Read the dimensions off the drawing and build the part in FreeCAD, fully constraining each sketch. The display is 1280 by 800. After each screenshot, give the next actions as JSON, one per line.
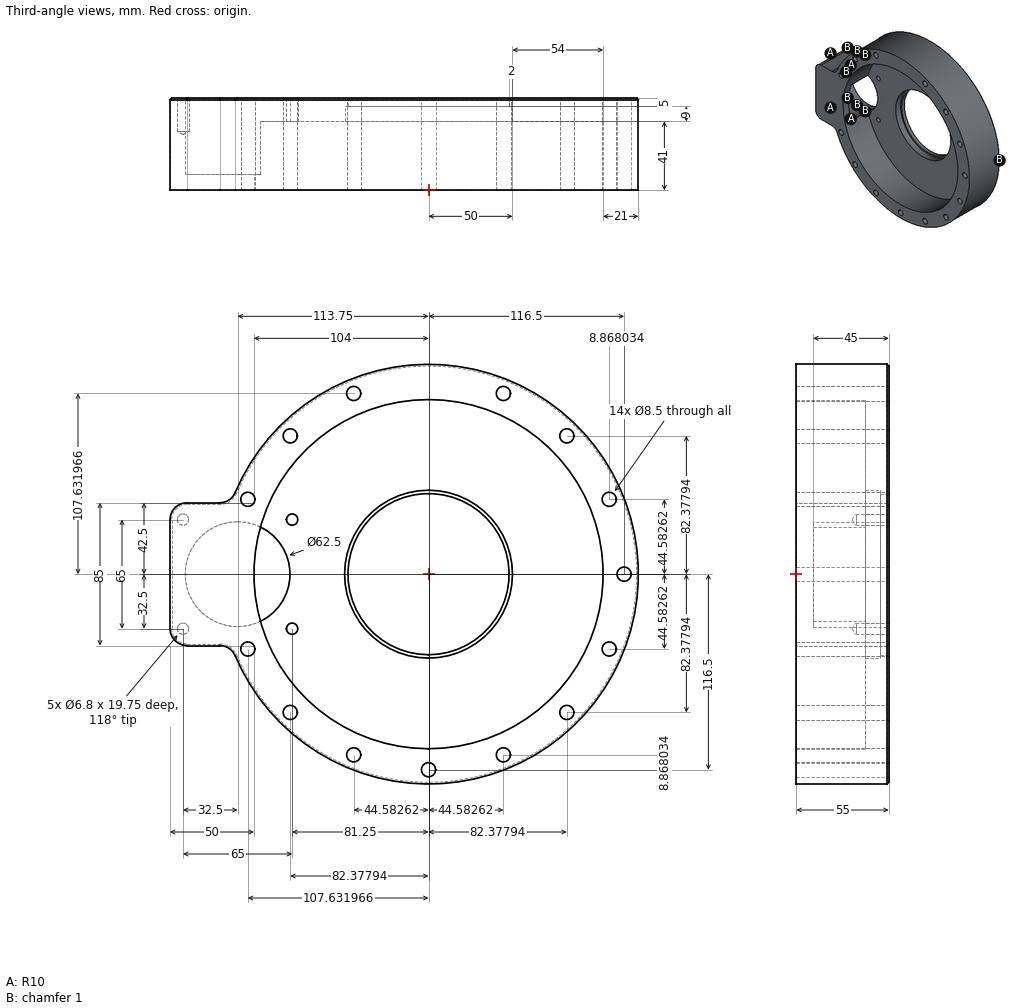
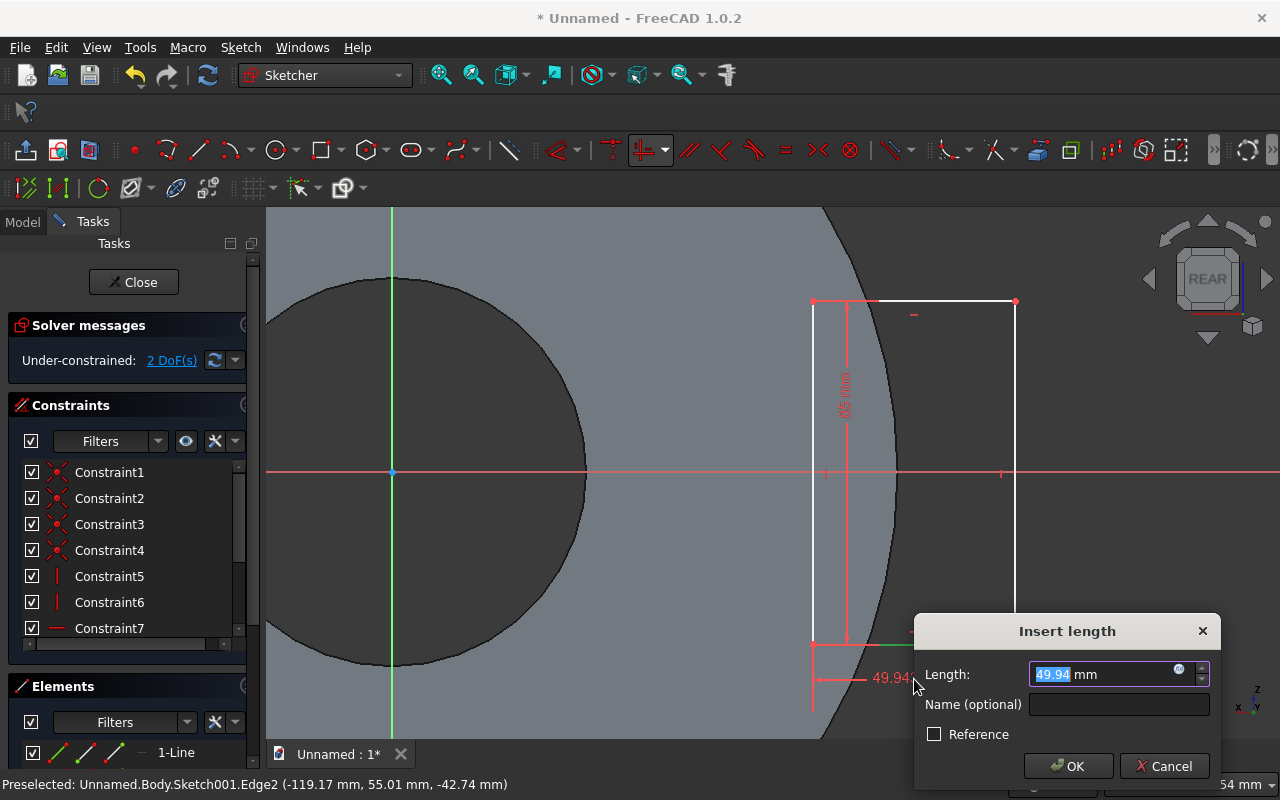
{"action": "type", "text": "50"}
{"action": "key", "text": "Return"}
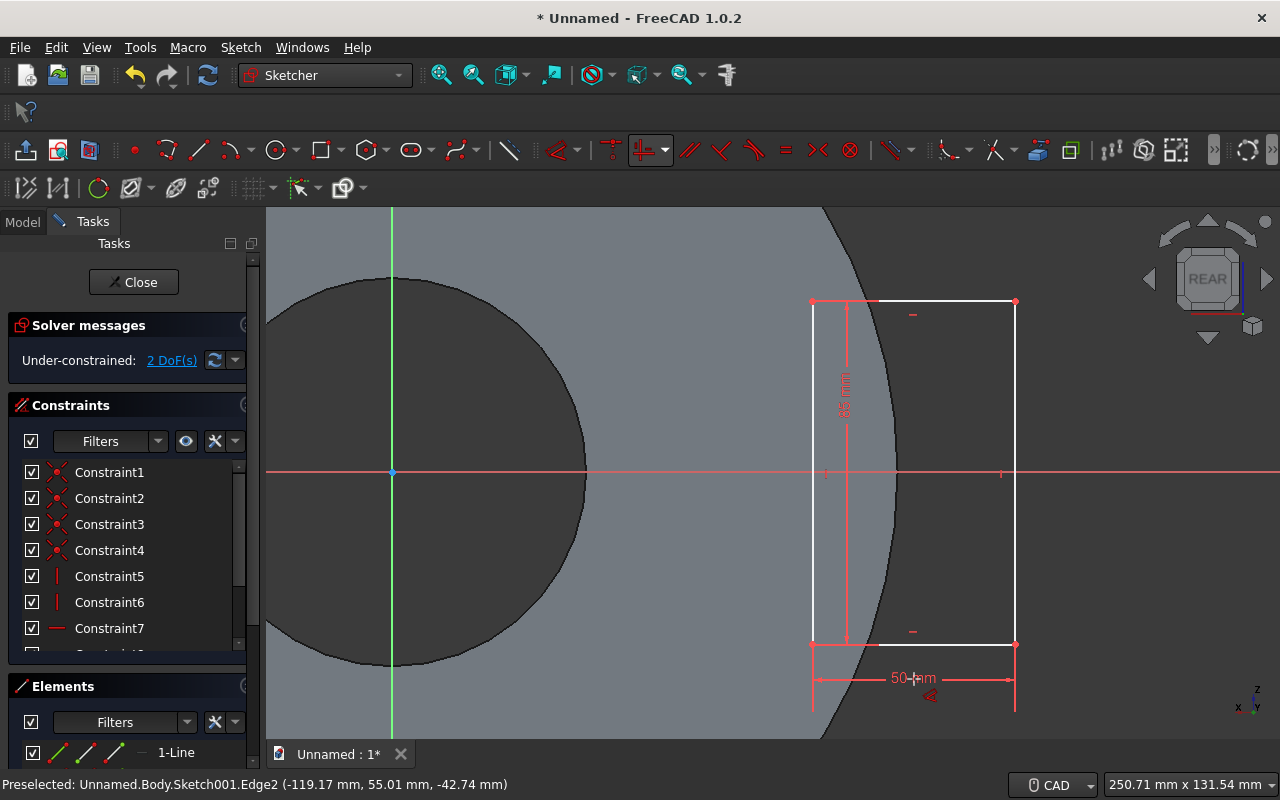
{"action": "left_click", "coordinate": [813, 301]}
{"action": "left_click", "coordinate": [602, 267]}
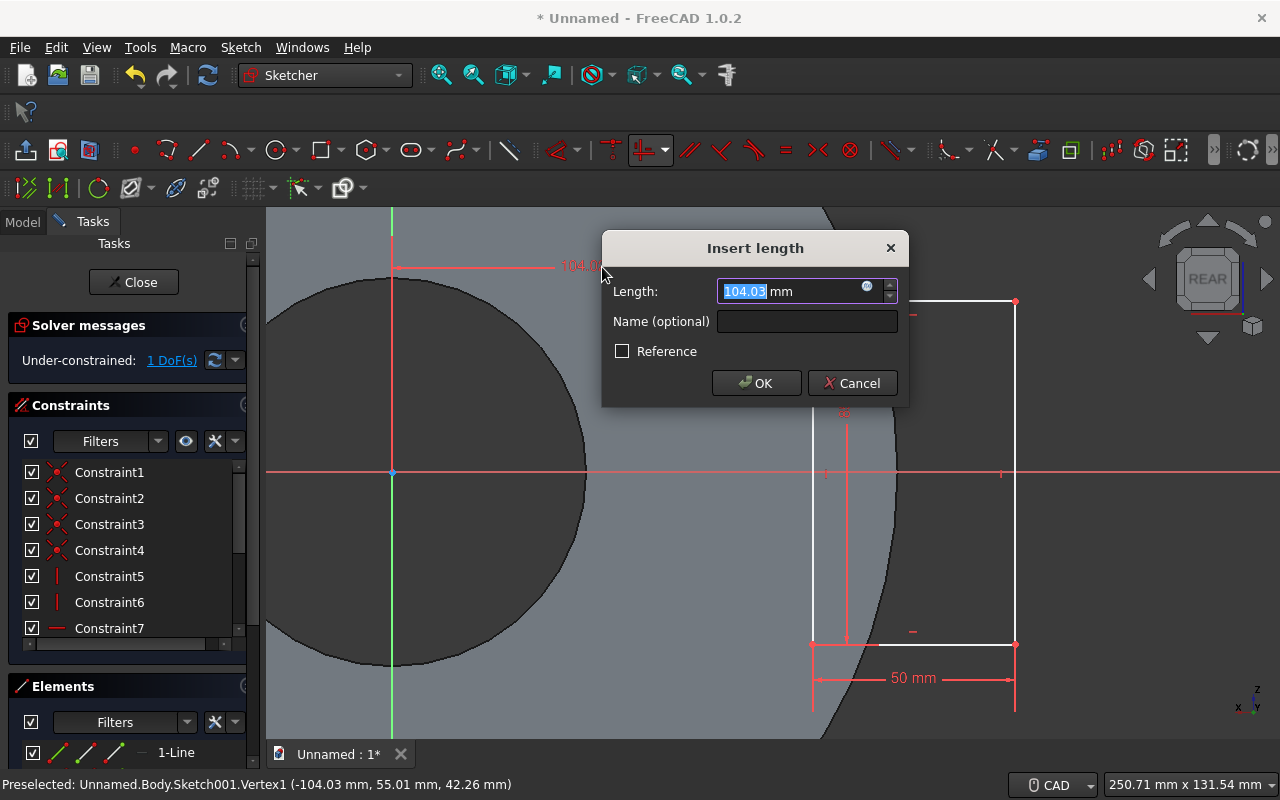
{"action": "type", "text": "104"}
{"action": "key", "text": "Return"}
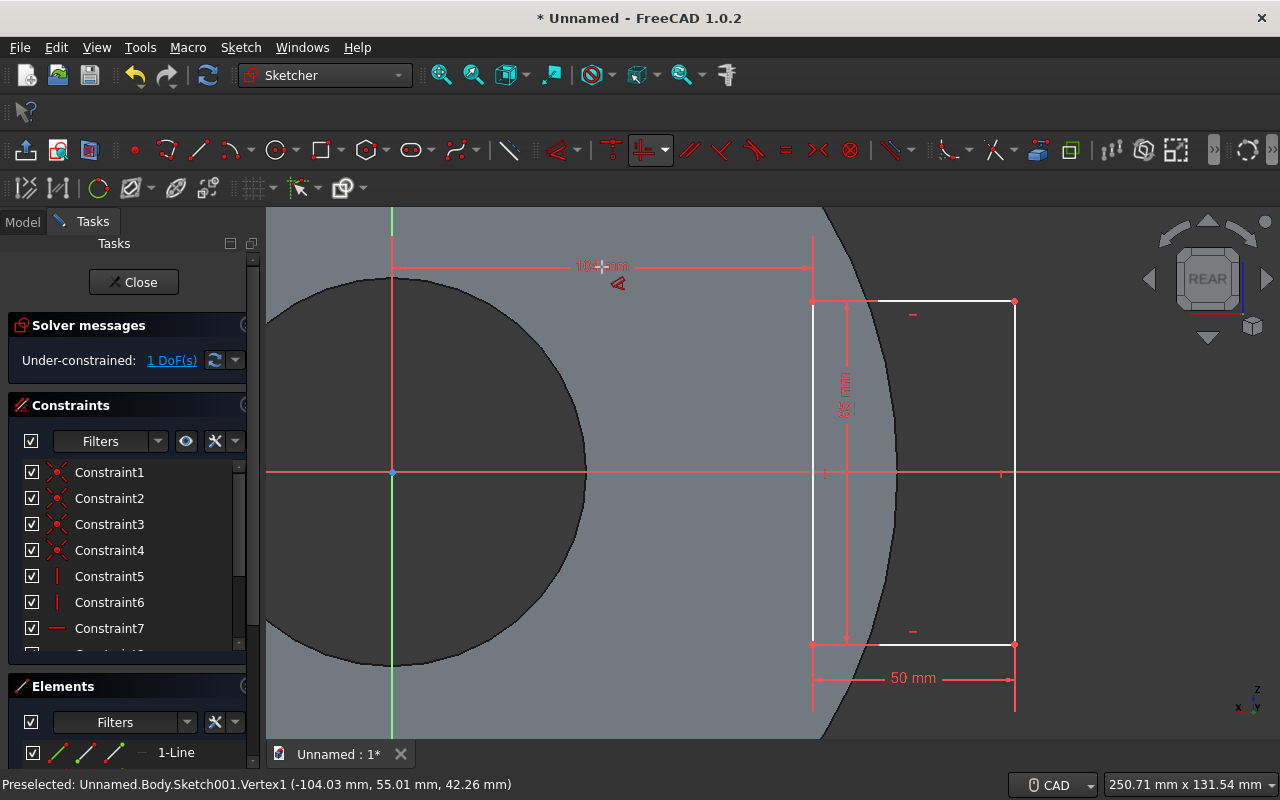
{"action": "left_click", "coordinate": [813, 301]}
{"action": "left_click", "coordinate": [358, 387]}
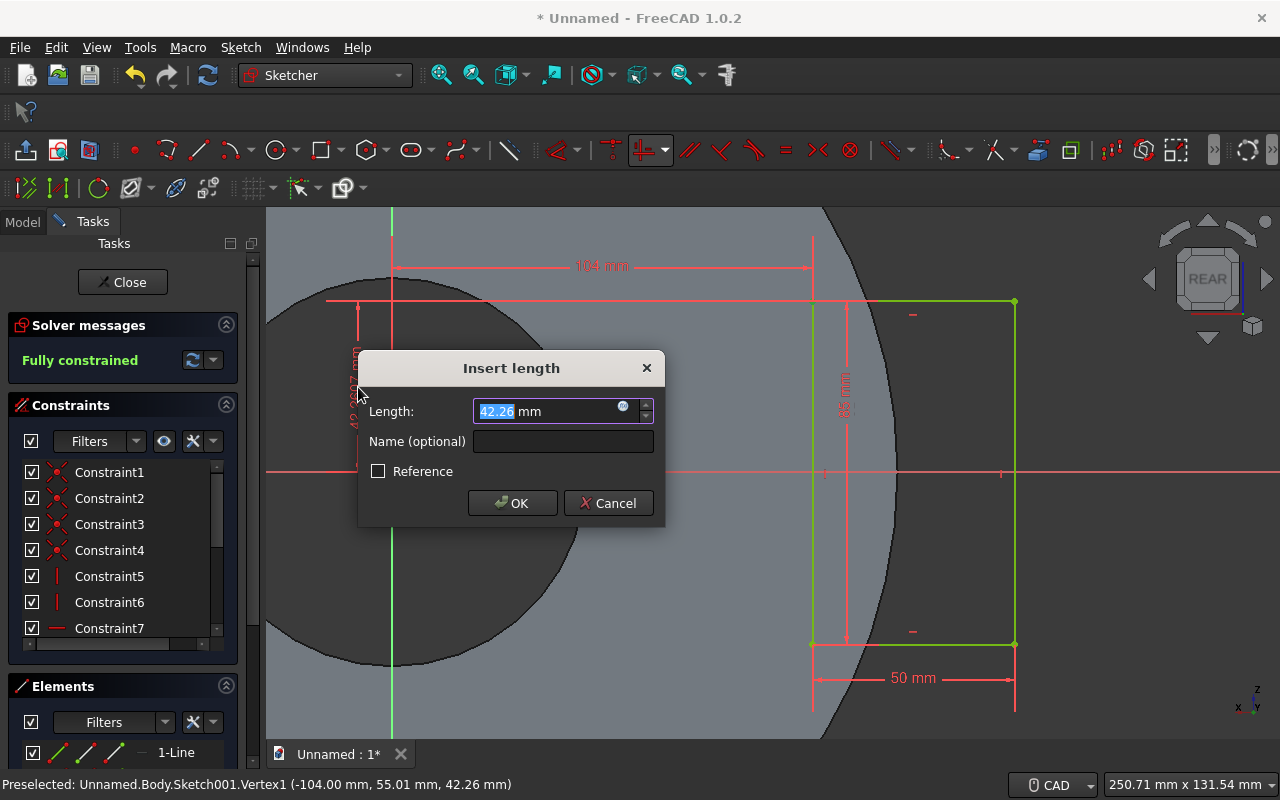
{"action": "type", "text": "42.5"}
{"action": "key", "text": "Return"}
{"action": "key", "text": "Escape"}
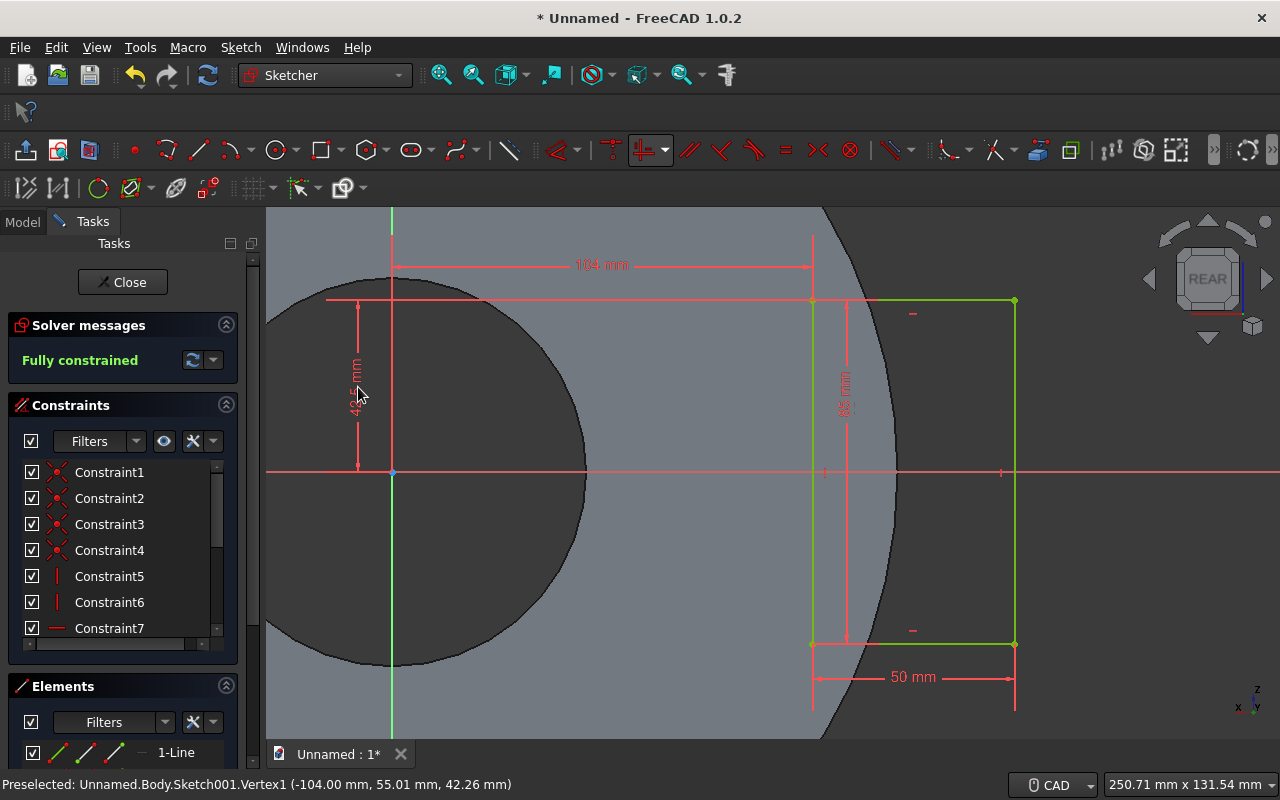
{"action": "left_click", "coordinate": [123, 282]}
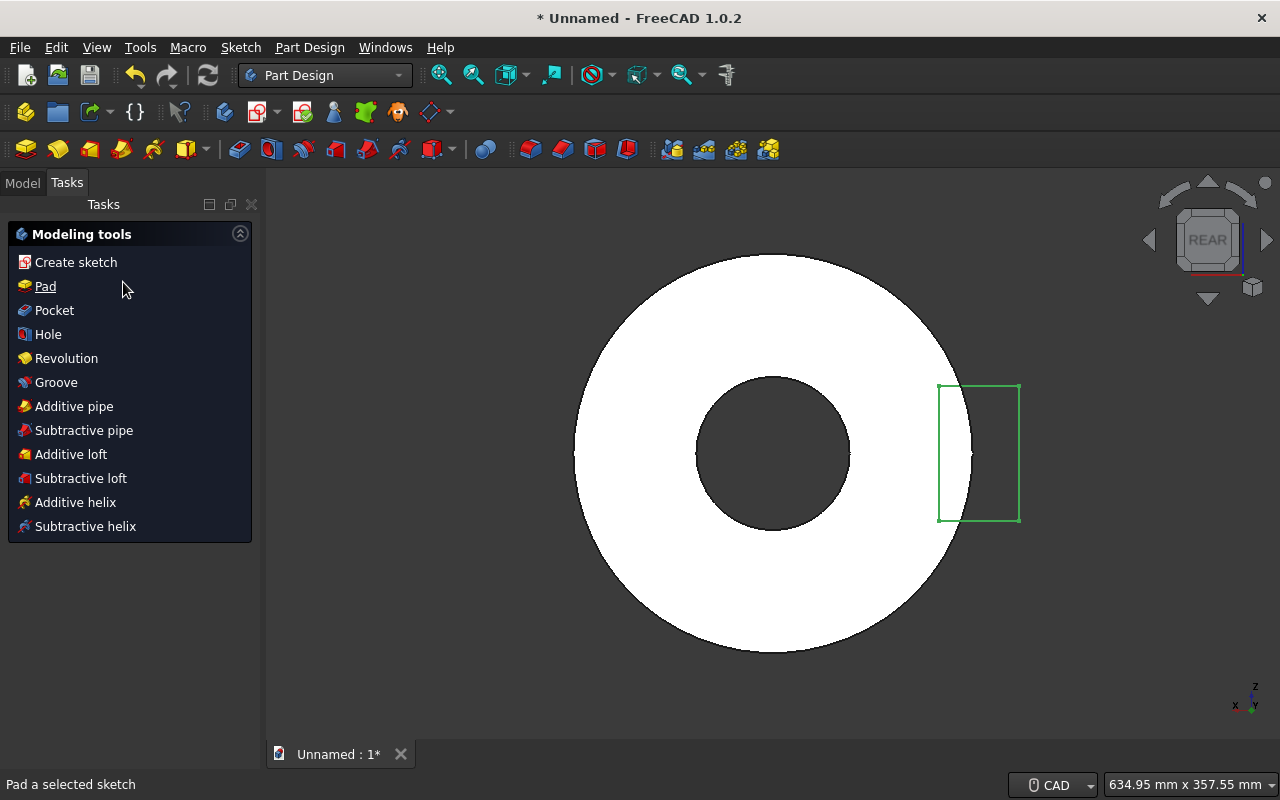
{"action": "left_click", "coordinate": [26, 150]}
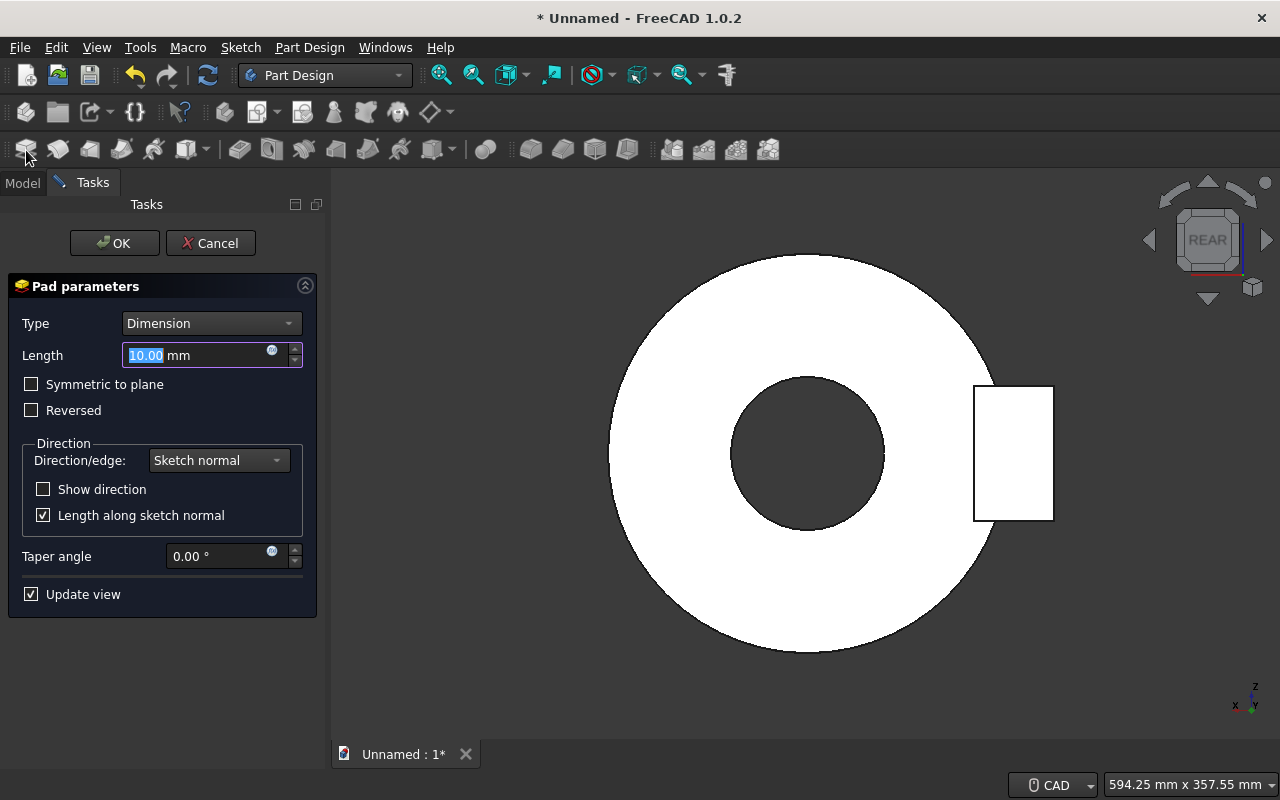
{"action": "type", "text": "55"}
{"action": "key", "text": "Tab"}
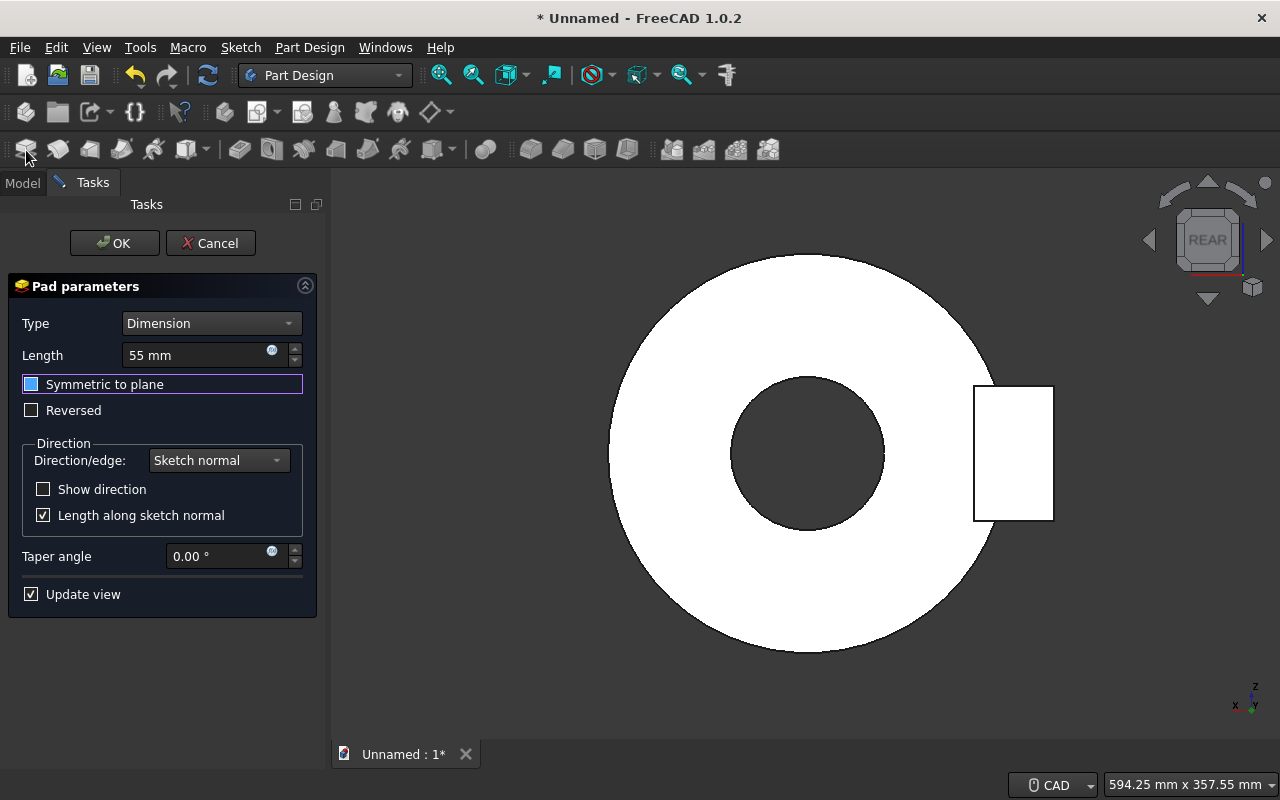
{"action": "left_click", "coordinate": [30, 410]}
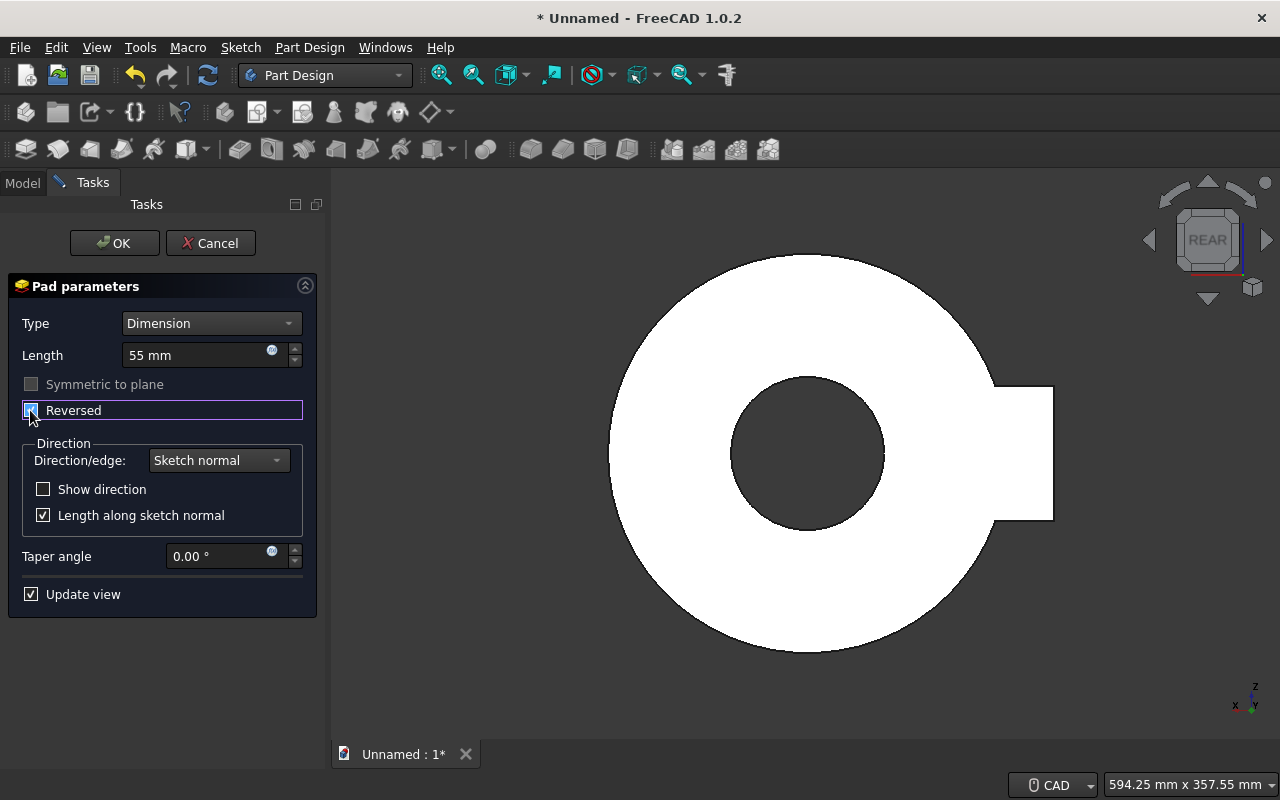
{"action": "left_click", "coordinate": [115, 243]}